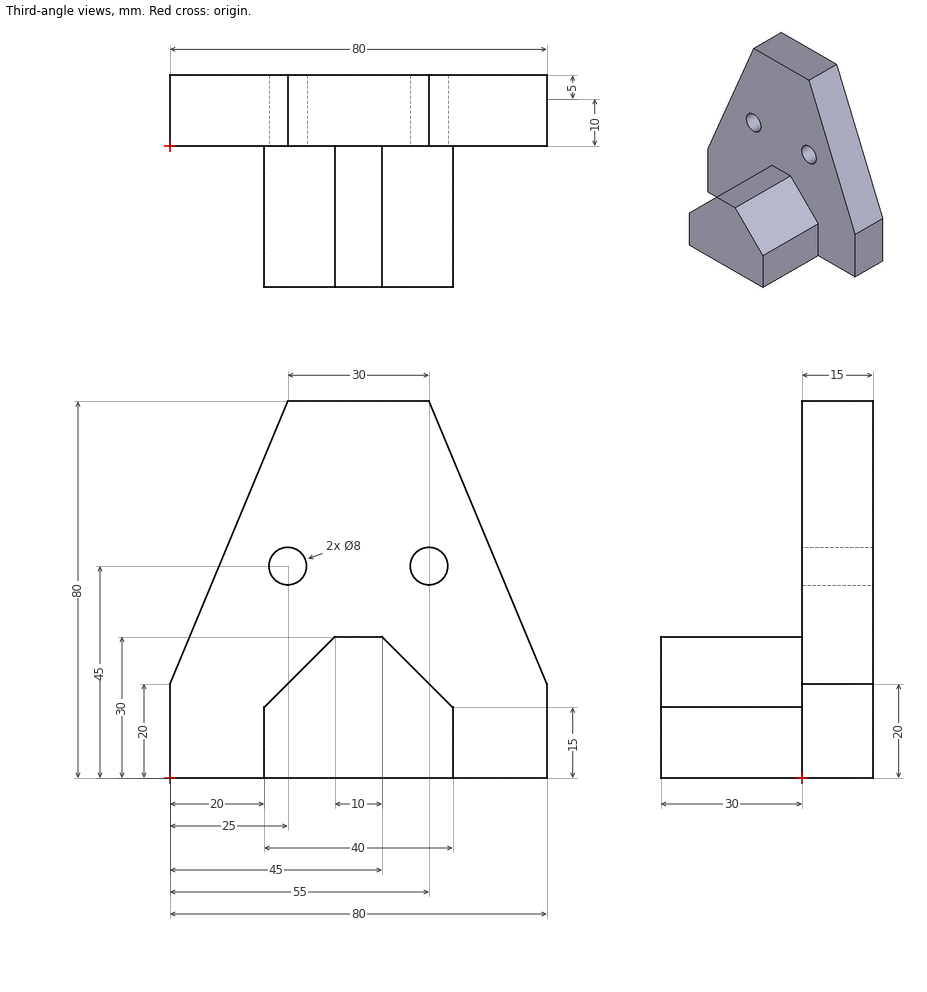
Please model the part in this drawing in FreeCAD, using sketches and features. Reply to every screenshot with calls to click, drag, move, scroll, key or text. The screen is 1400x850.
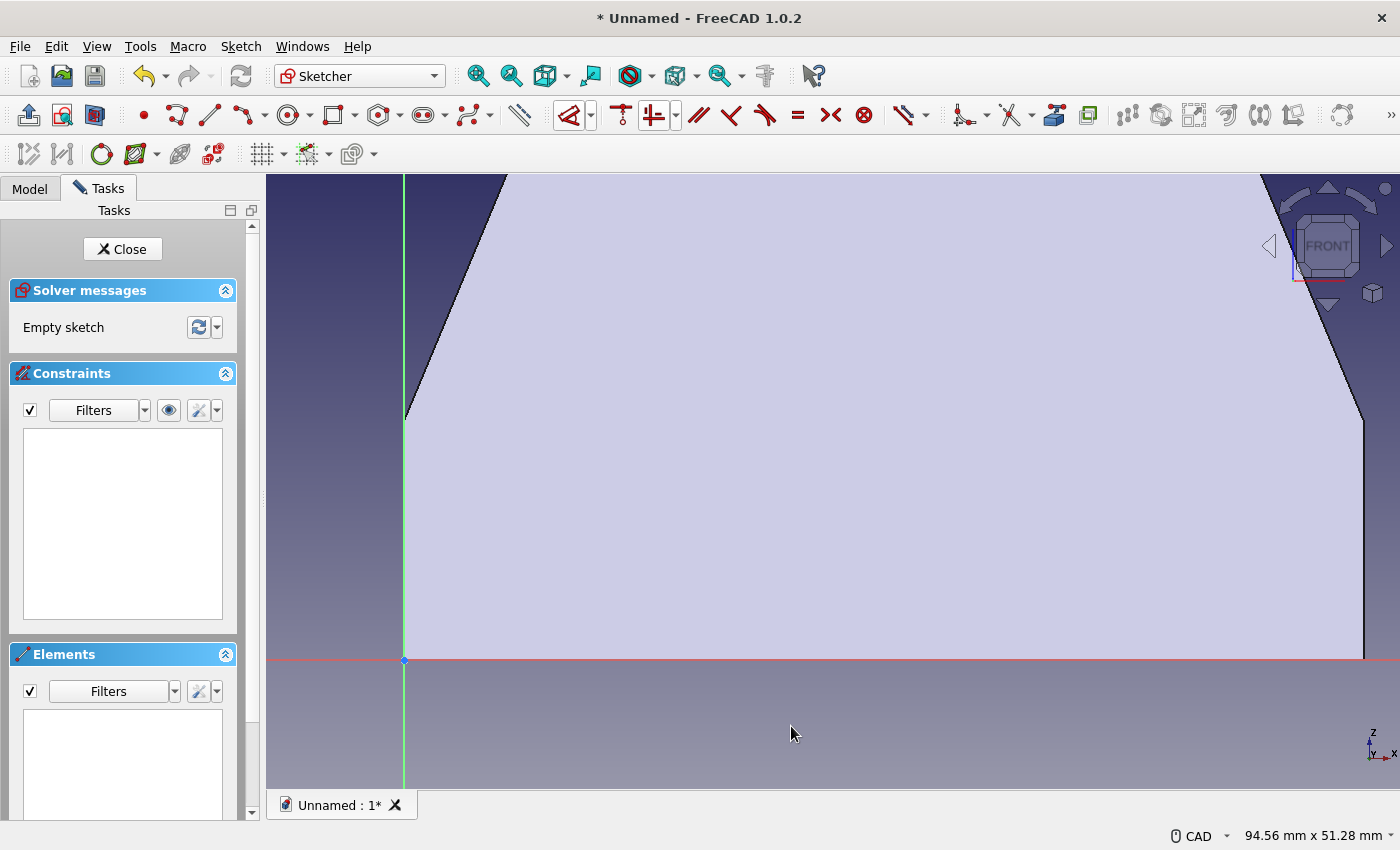
click(177, 116)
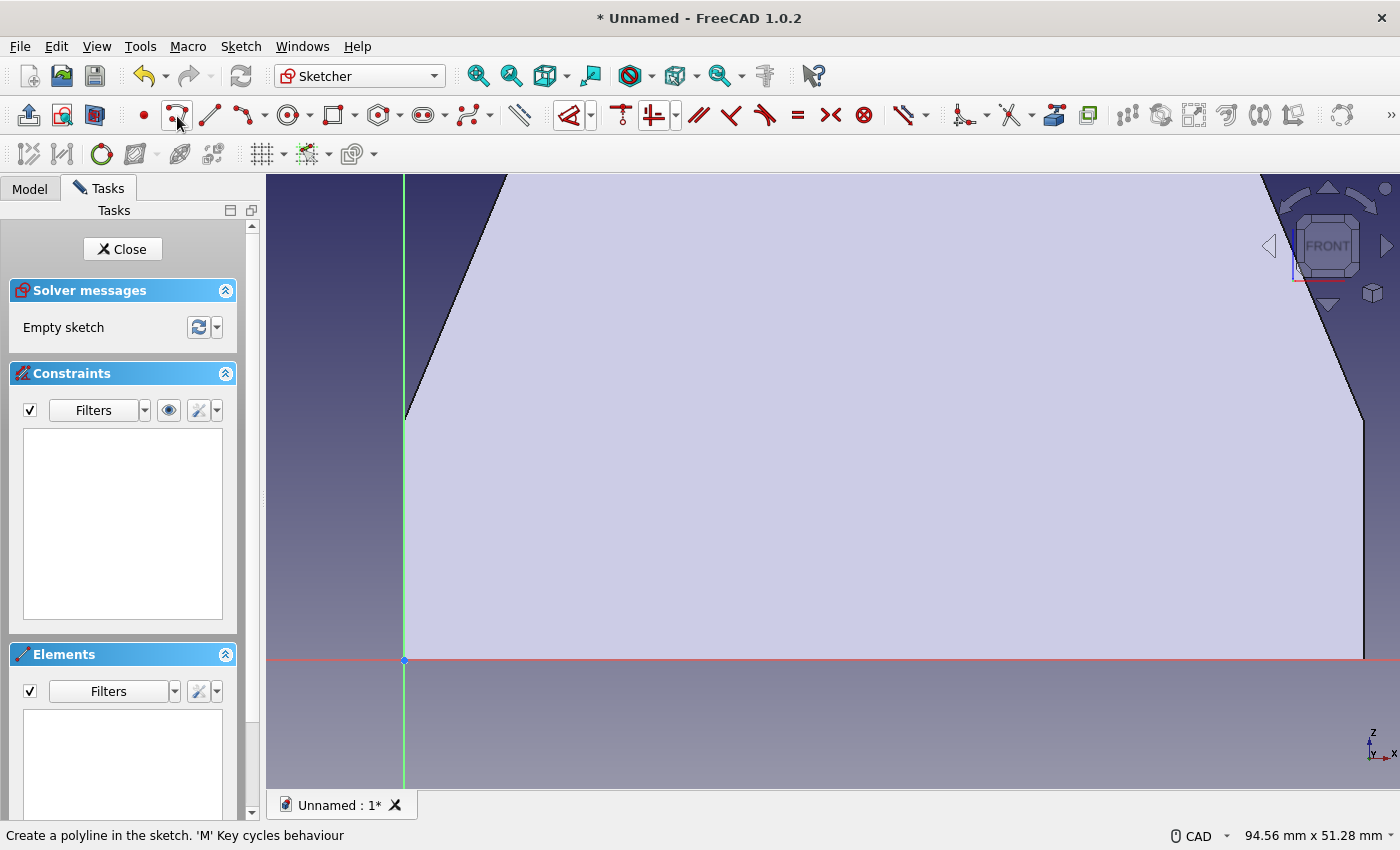
click(644, 660)
click(1124, 651)
click(1124, 481)
click(944, 301)
click(824, 301)
click(644, 481)
click(644, 660)
key(Escape)
key(Escape)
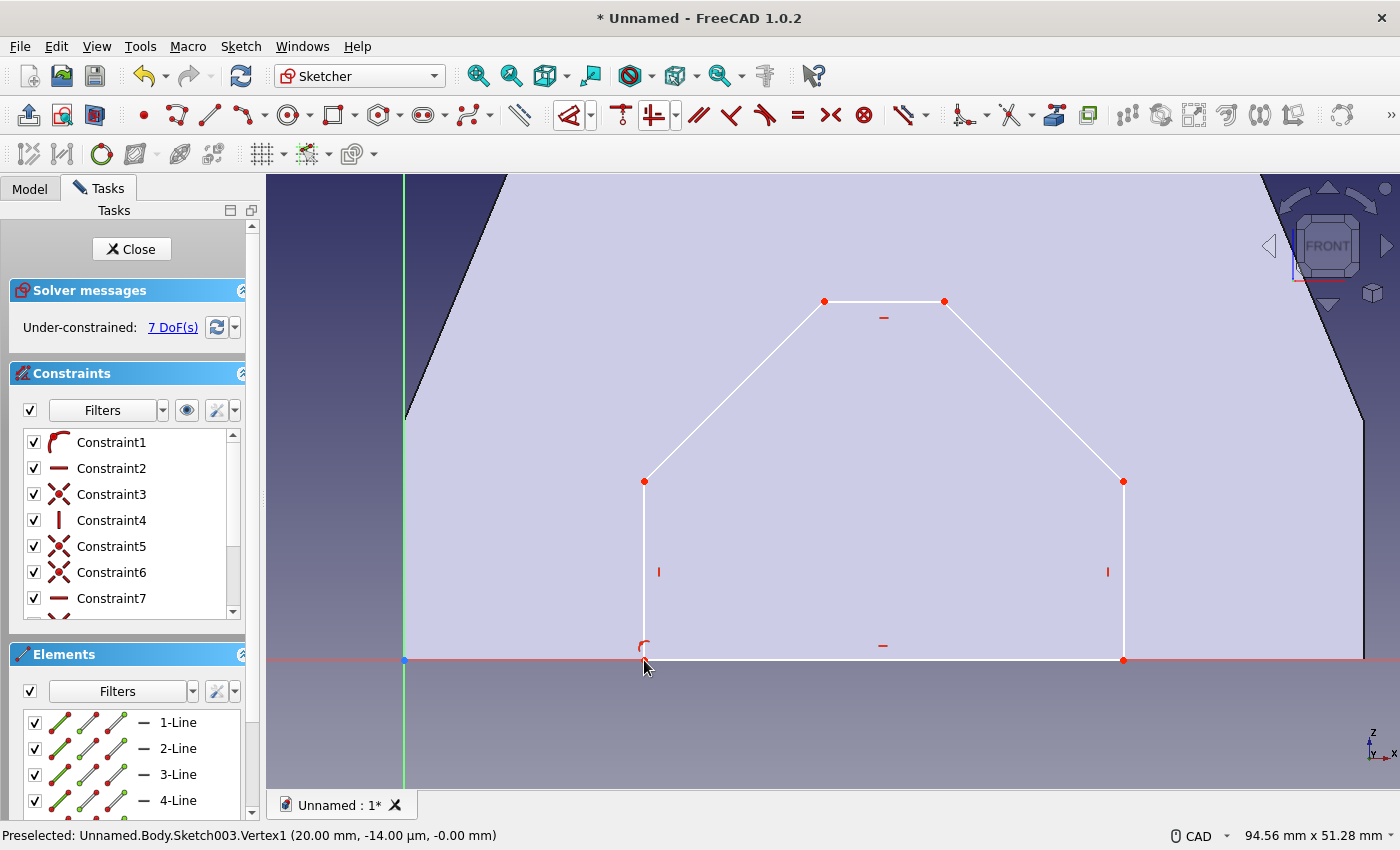
click(788, 660)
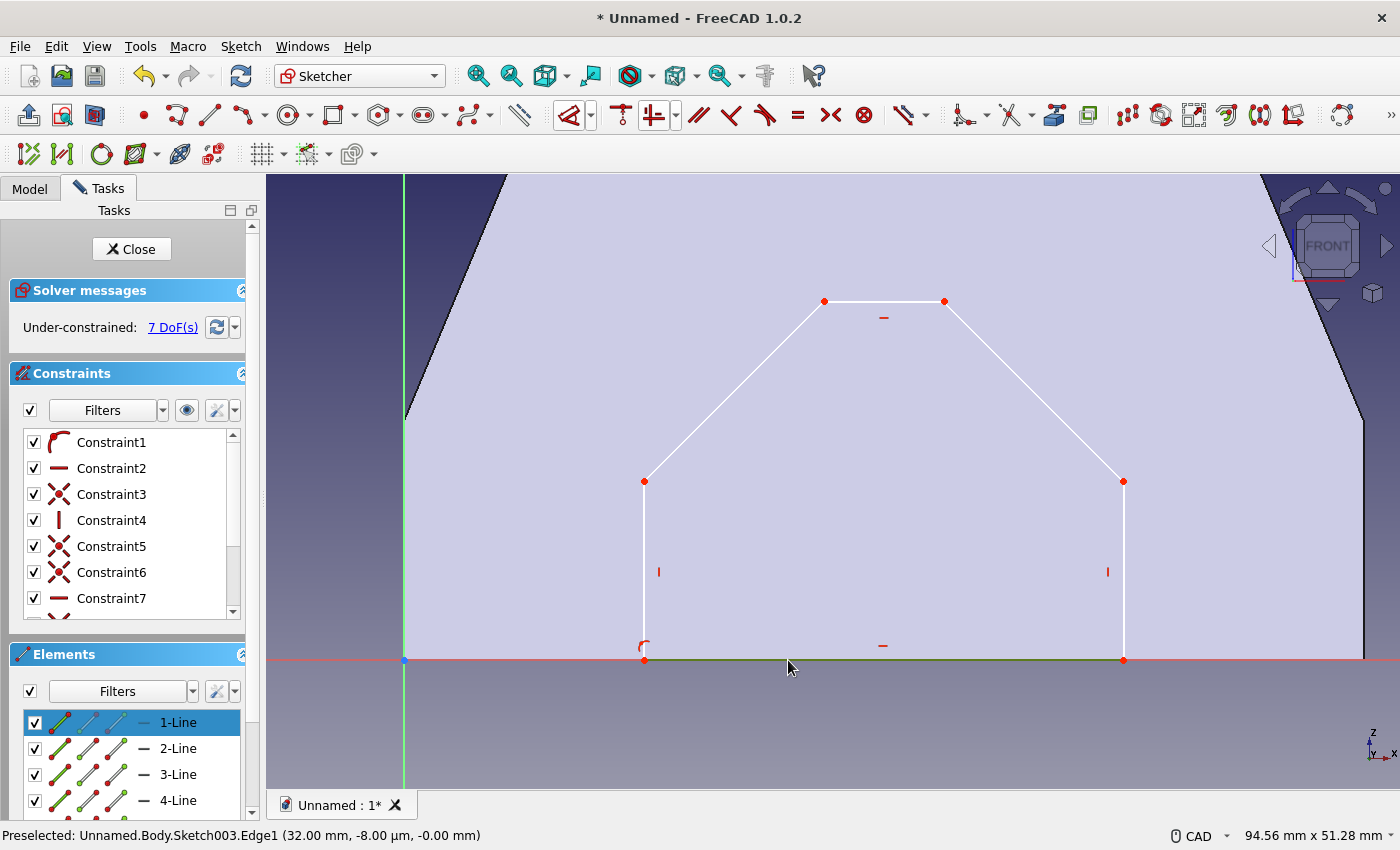
click(590, 116)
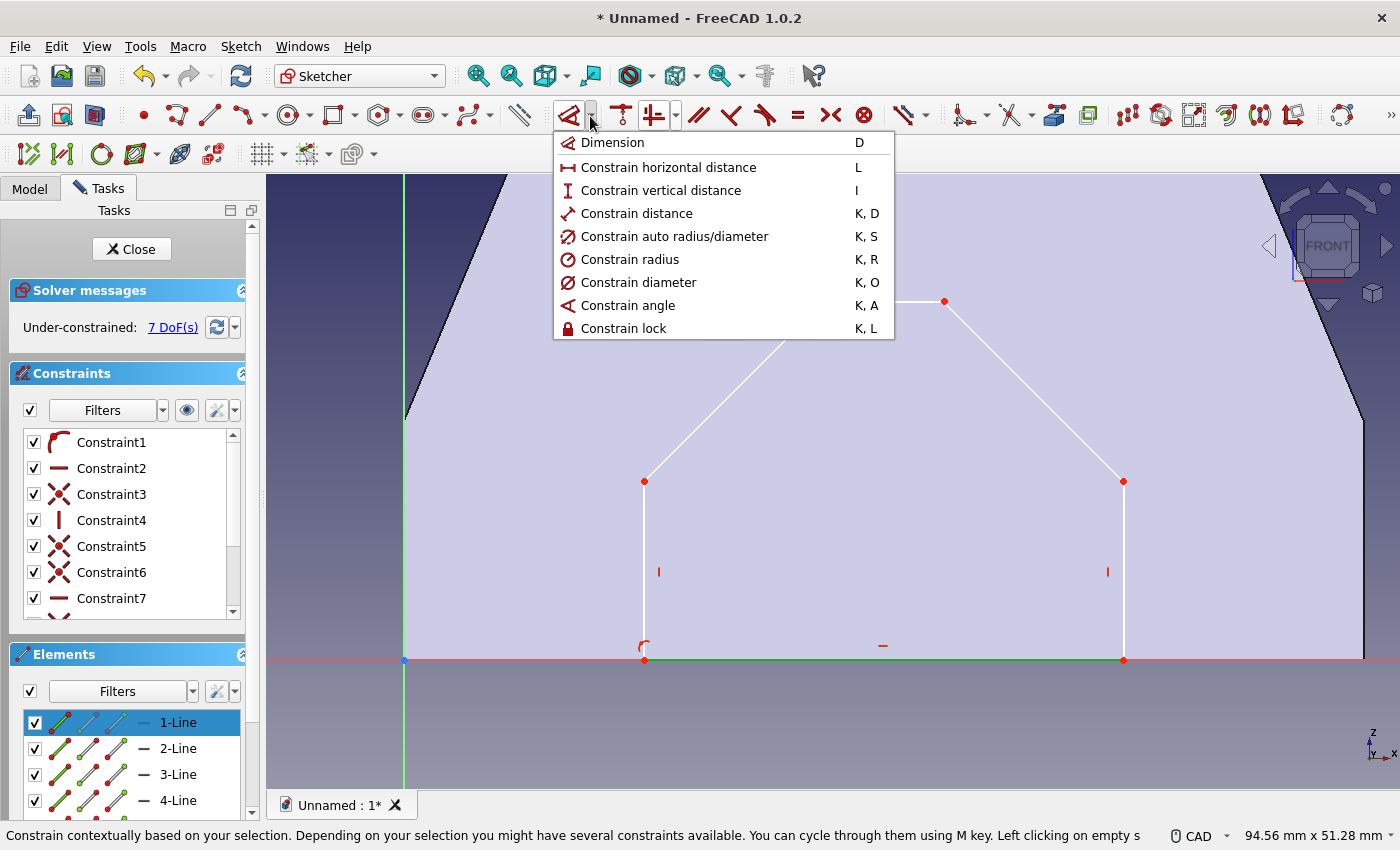
click(724, 168)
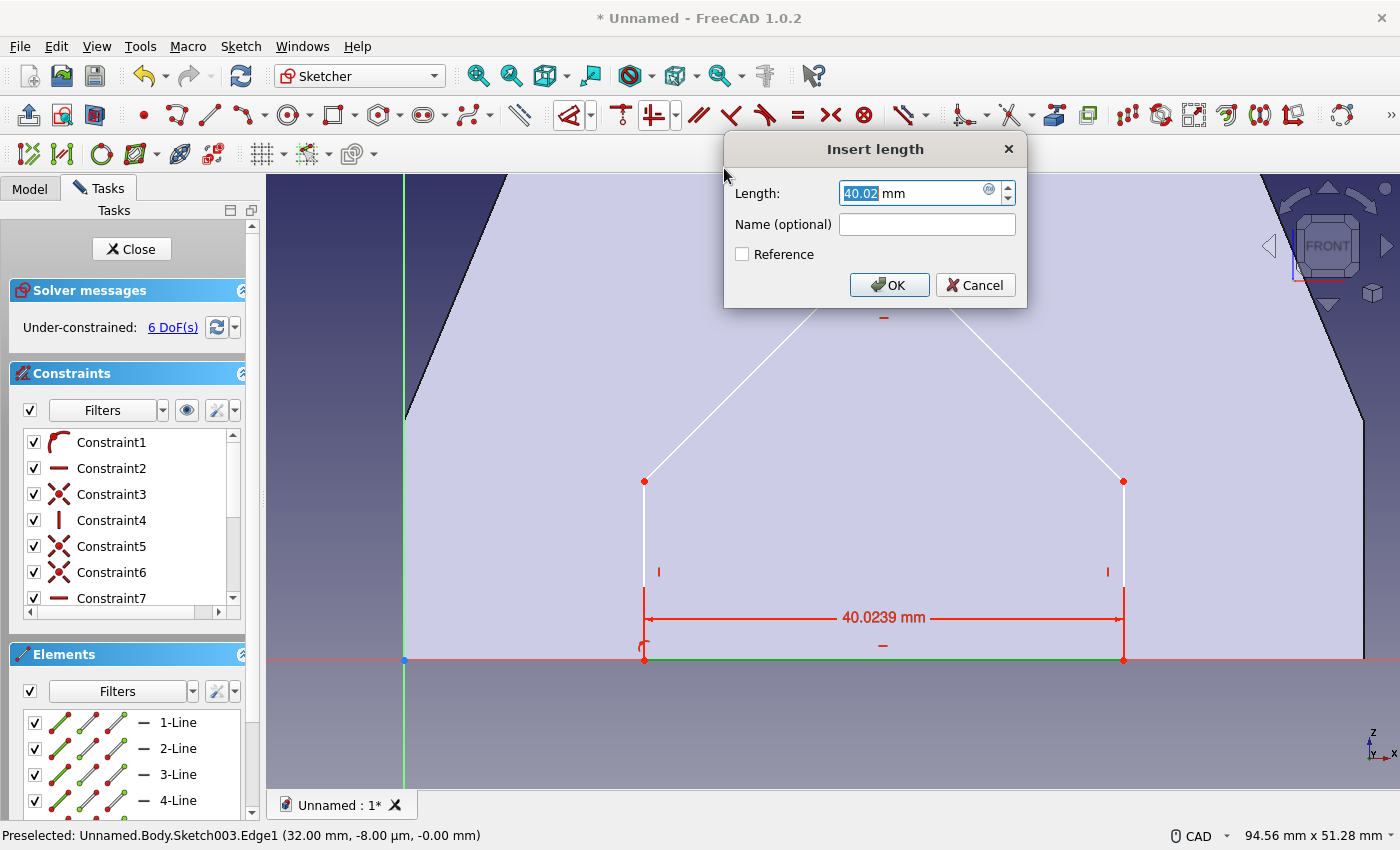
text(40)
key(Return)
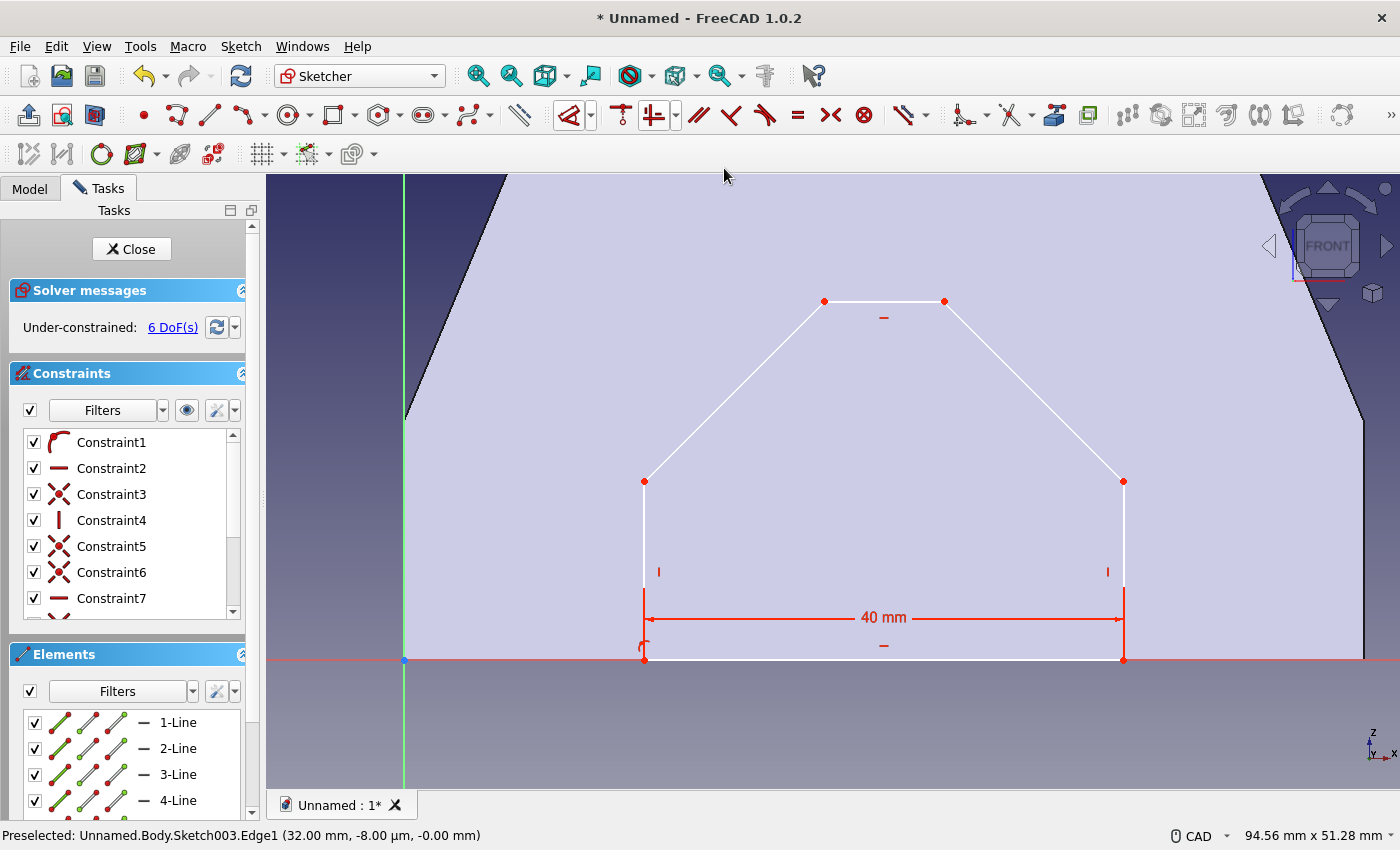
click(1124, 607)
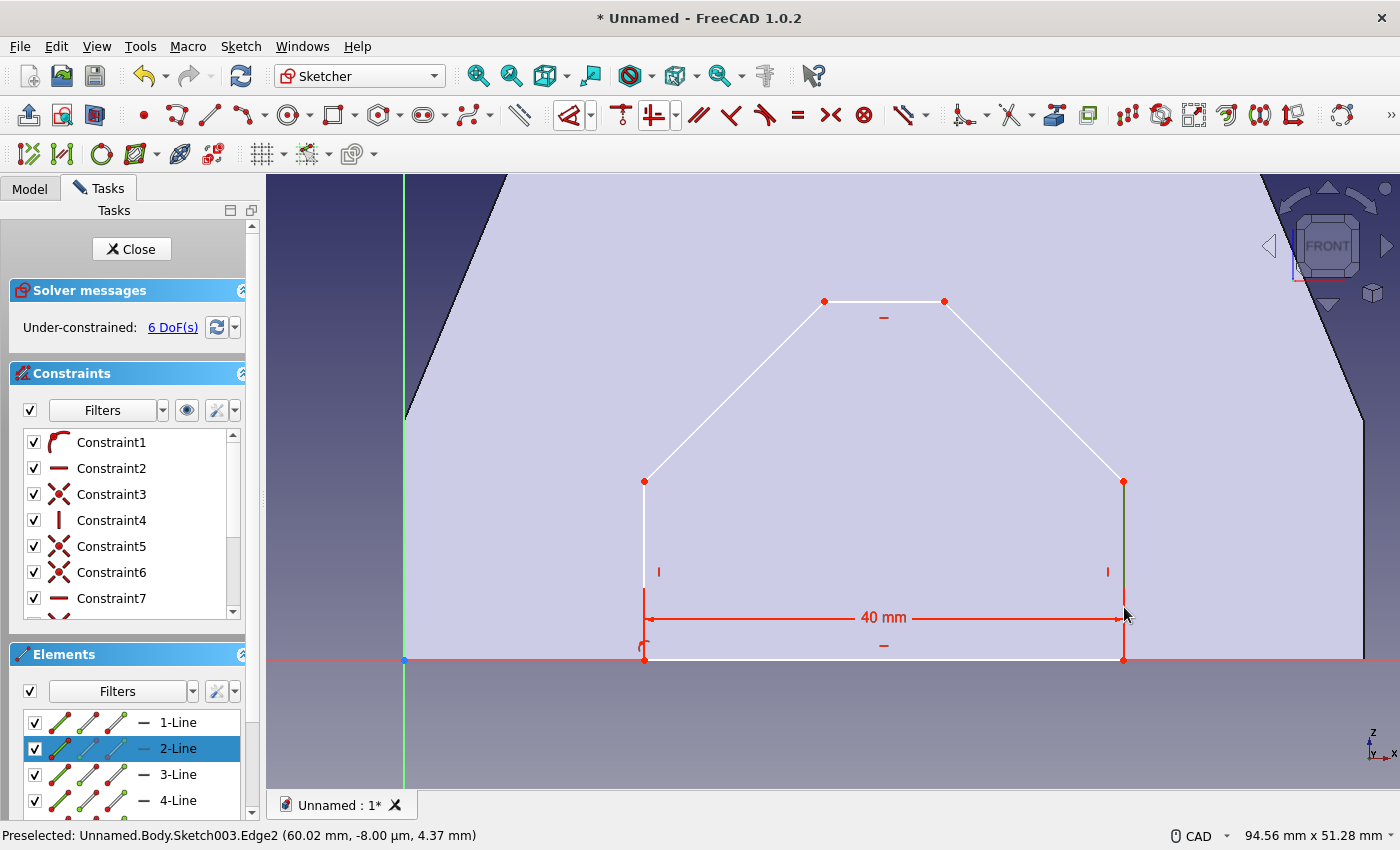
key(i)